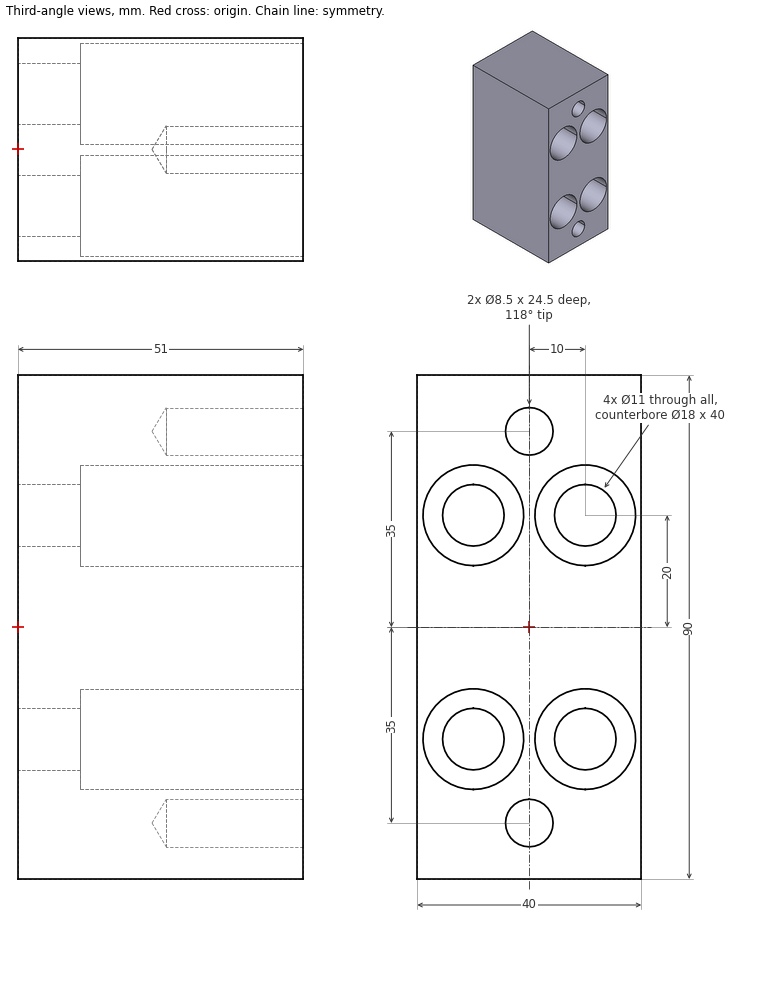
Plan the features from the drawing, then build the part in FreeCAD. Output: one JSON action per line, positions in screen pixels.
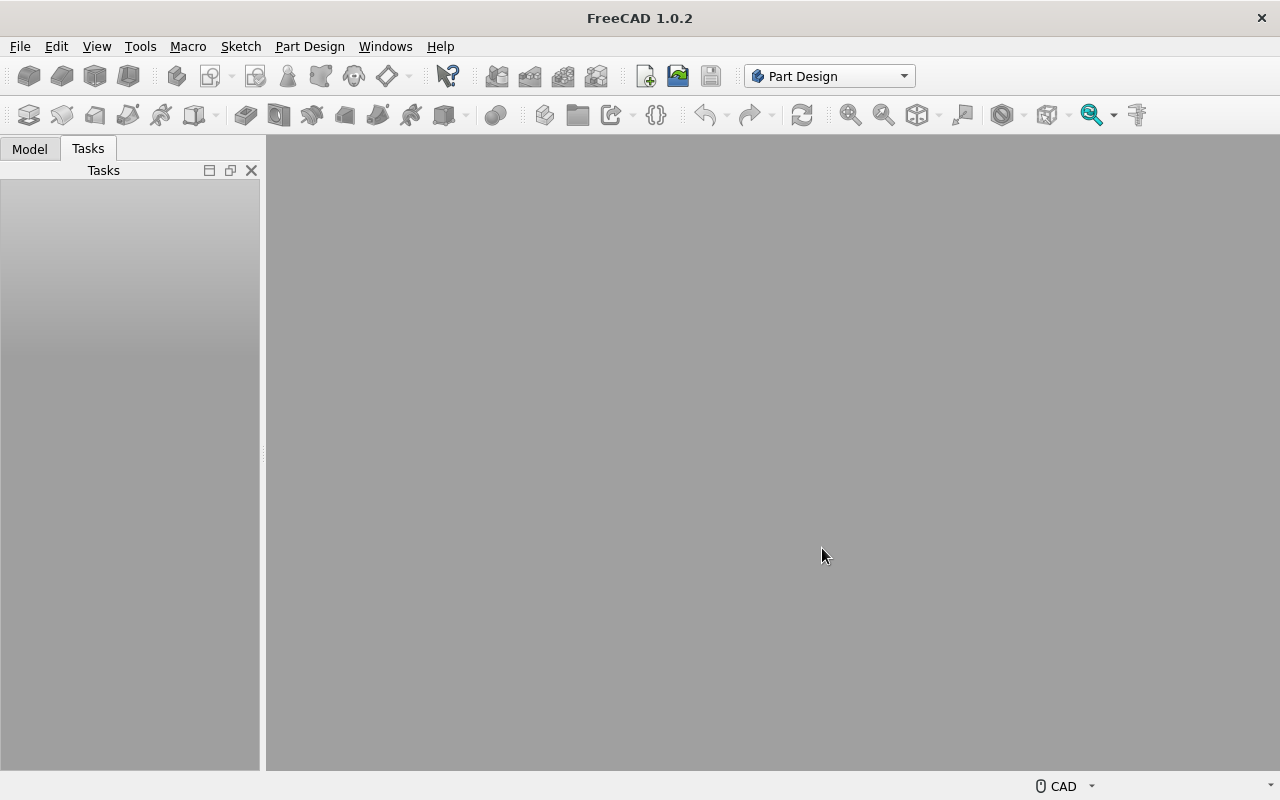
{"action": "left_click", "coordinate": [645, 76]}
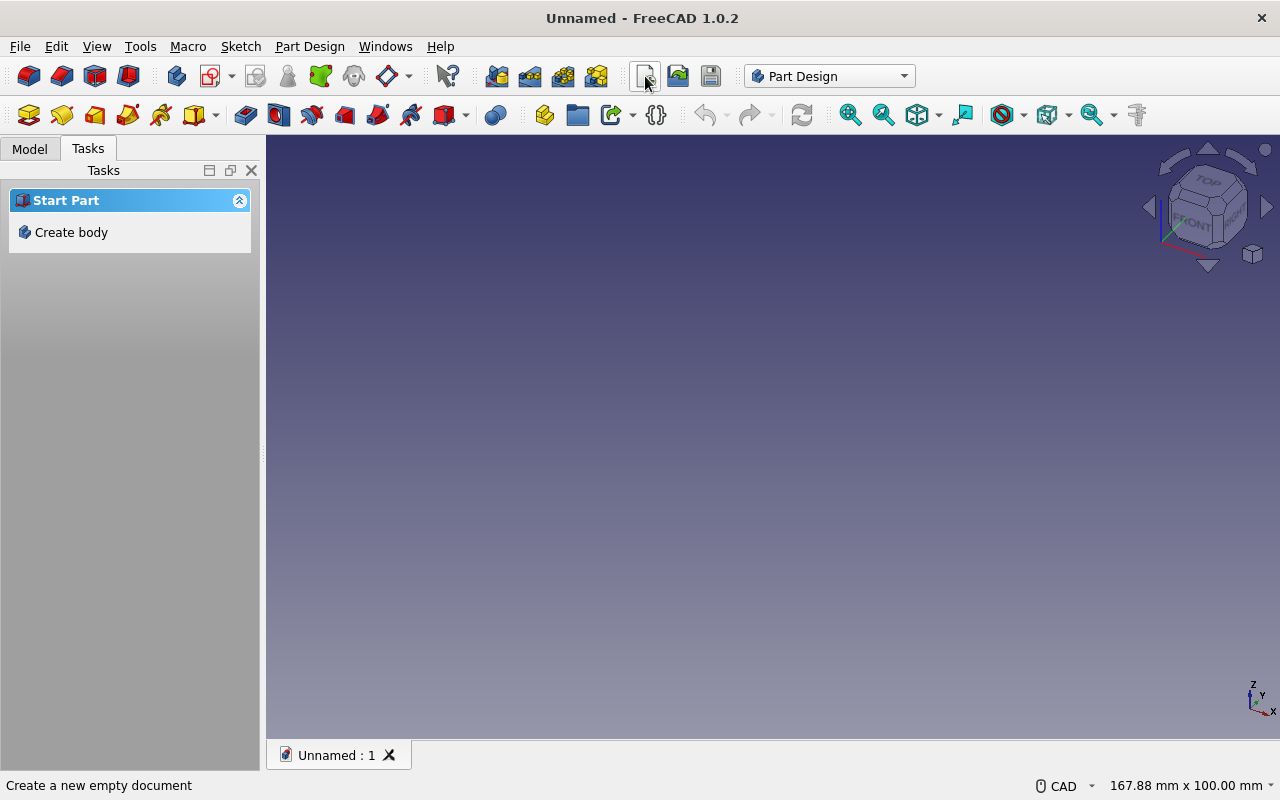
{"action": "left_click", "coordinate": [210, 76]}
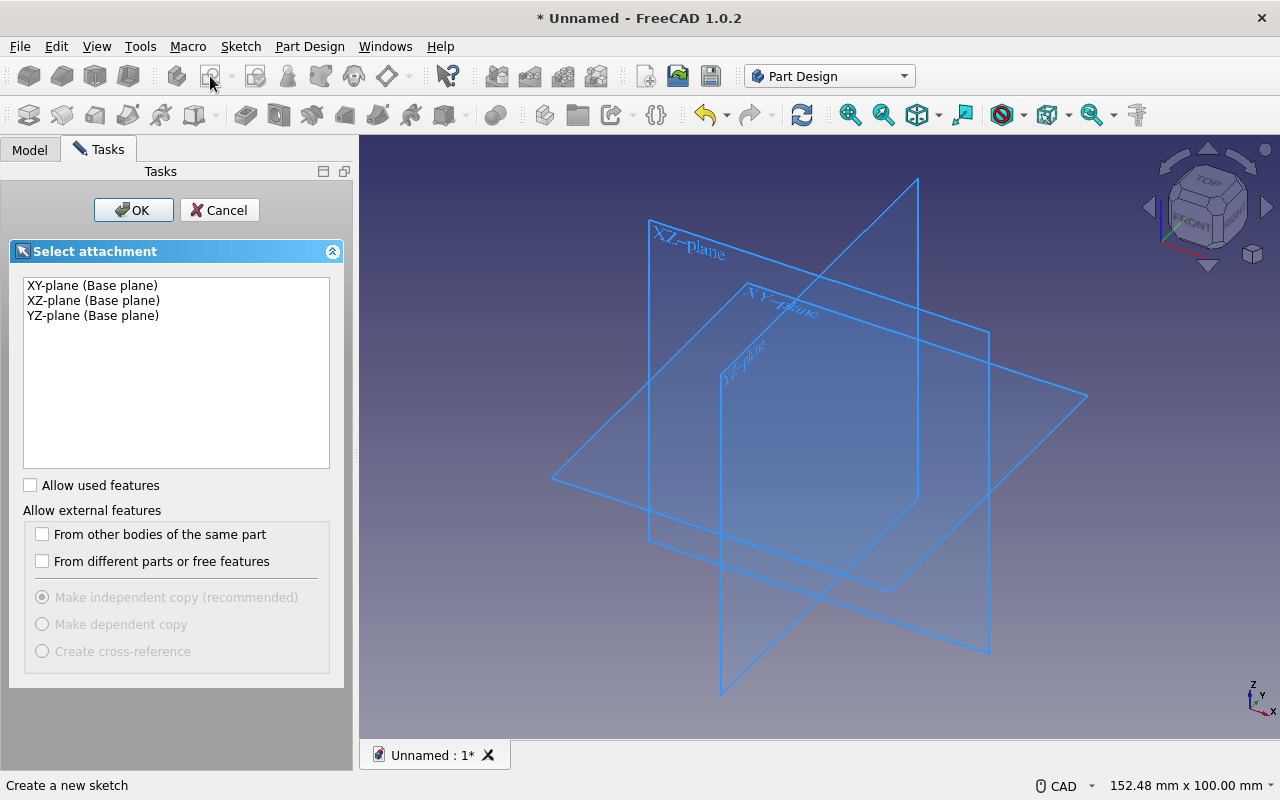
{"action": "left_click", "coordinate": [84, 316]}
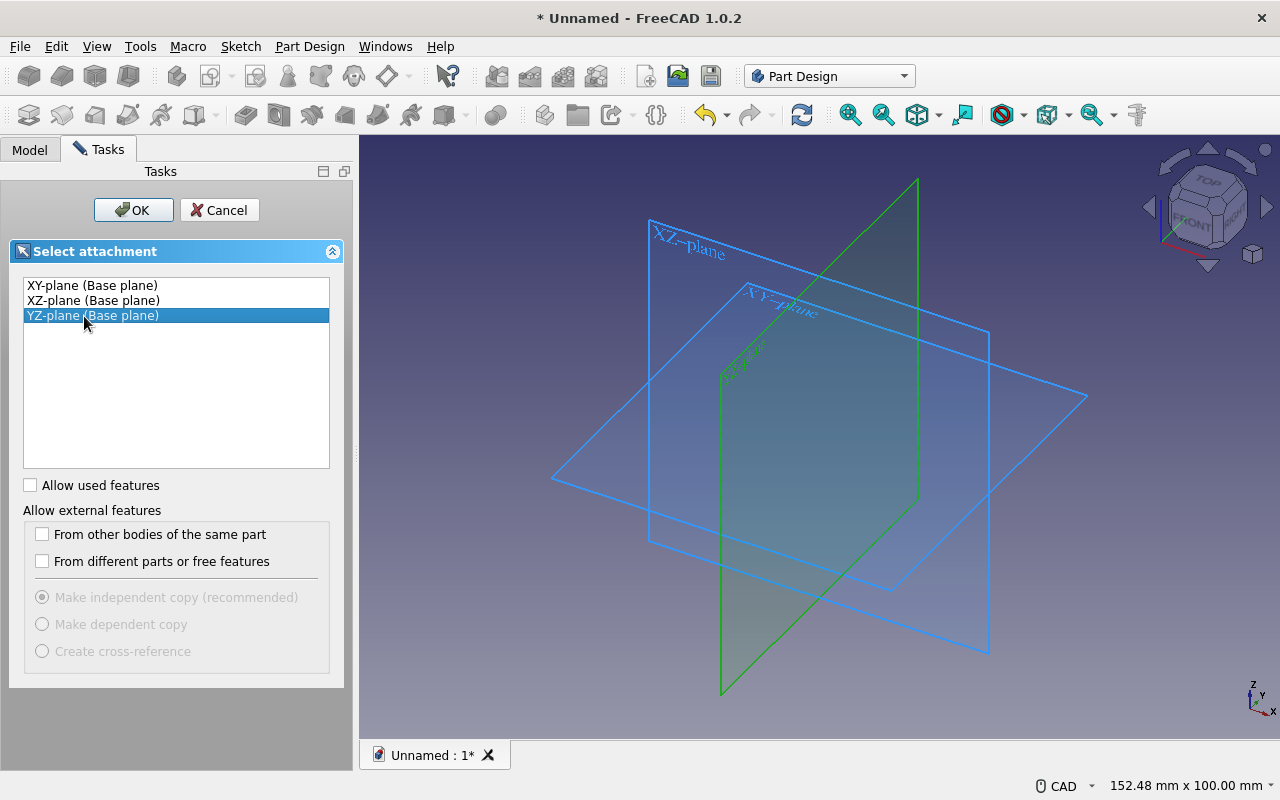
{"action": "left_click", "coordinate": [134, 210]}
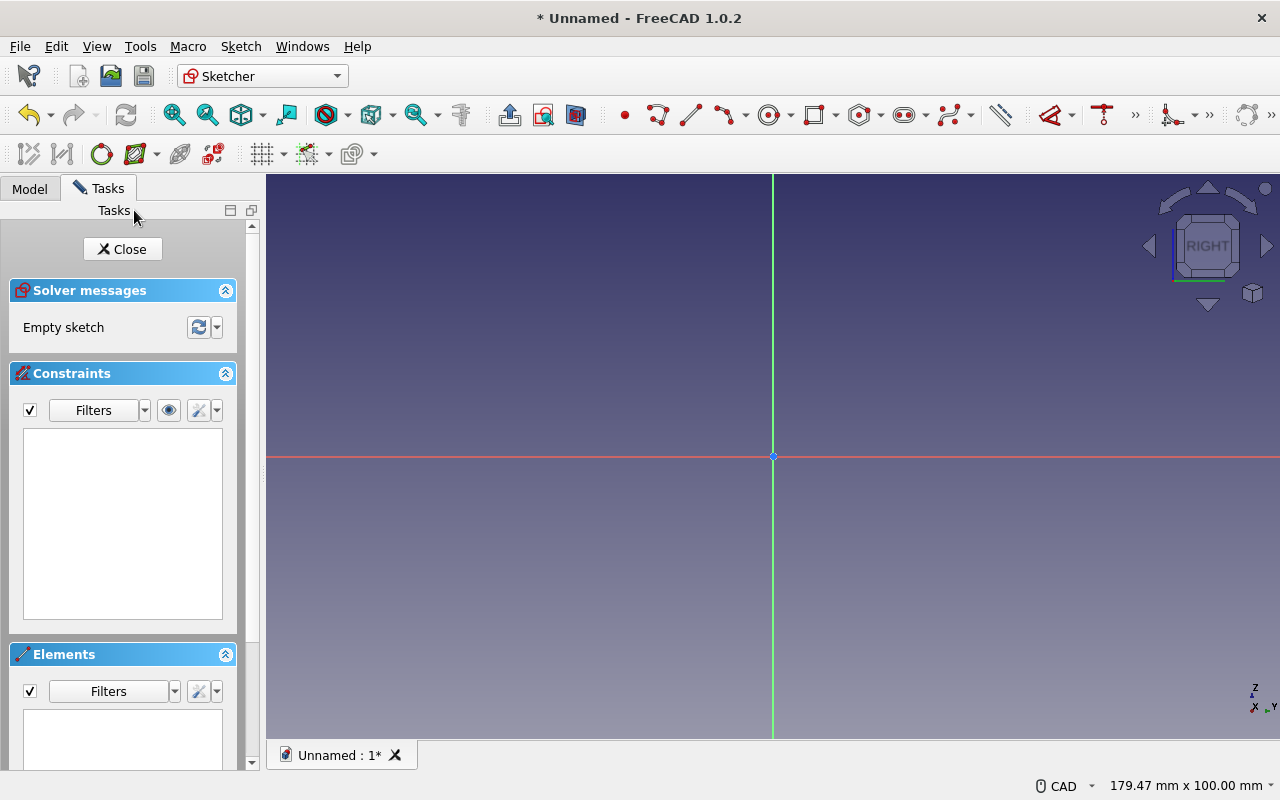
{"action": "scroll", "coordinate": [565, 457], "scroll_direction": "down", "scroll_amount": 2}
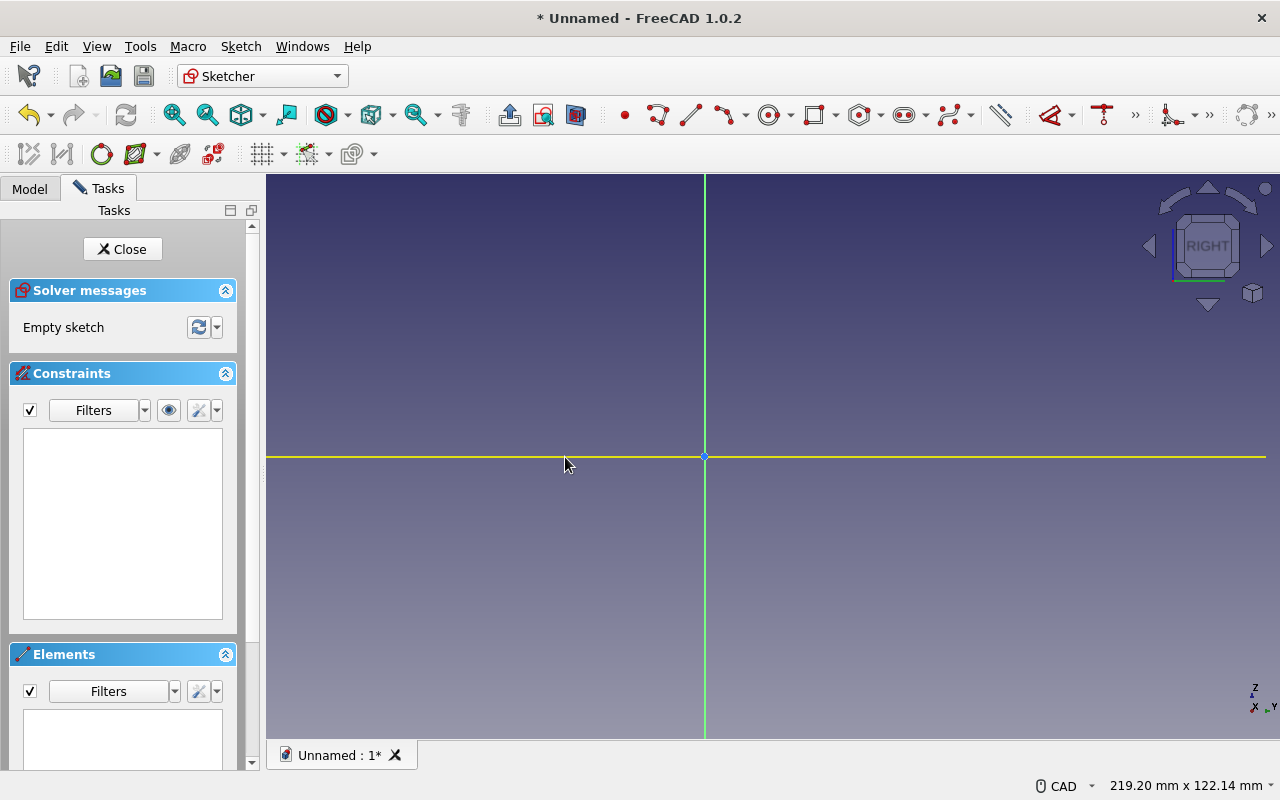
{"action": "key", "text": "g v"}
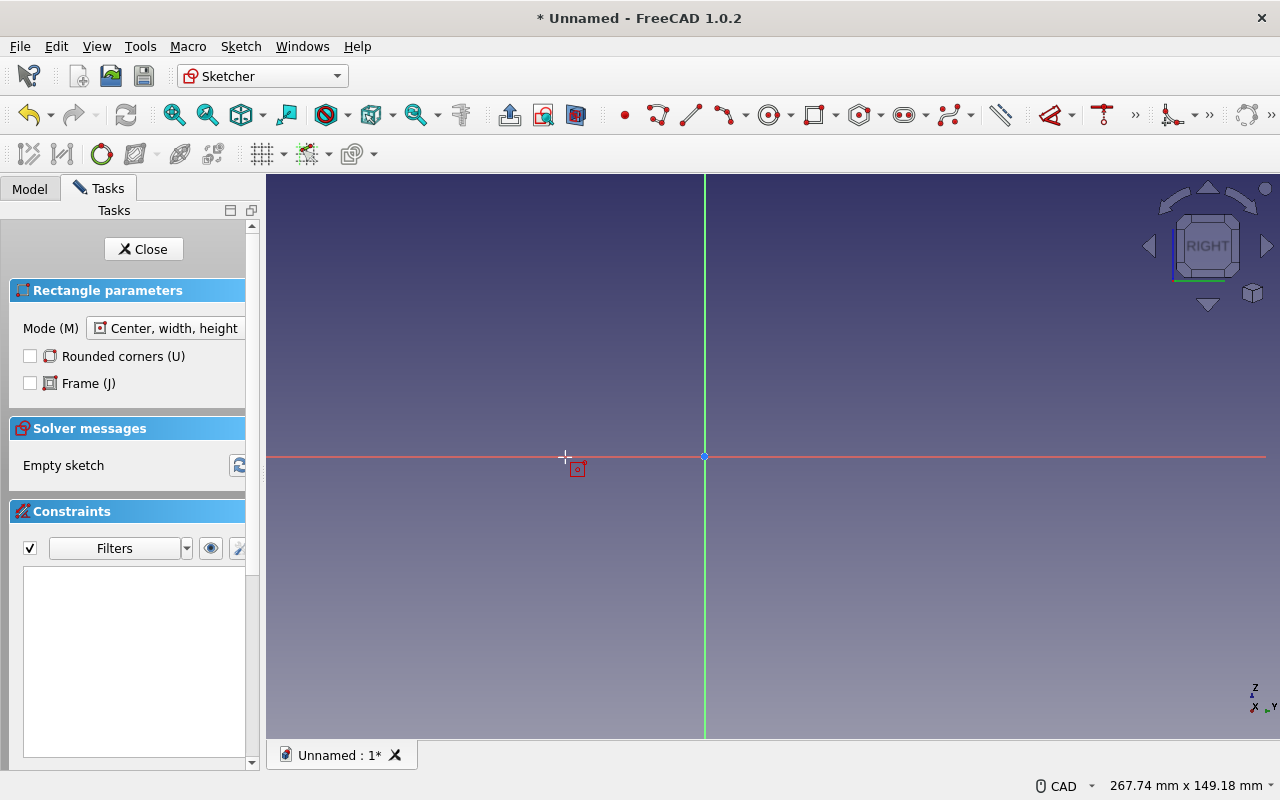
{"action": "left_click", "coordinate": [705, 457]}
{"action": "mouse_move", "coordinate": [780, 286]}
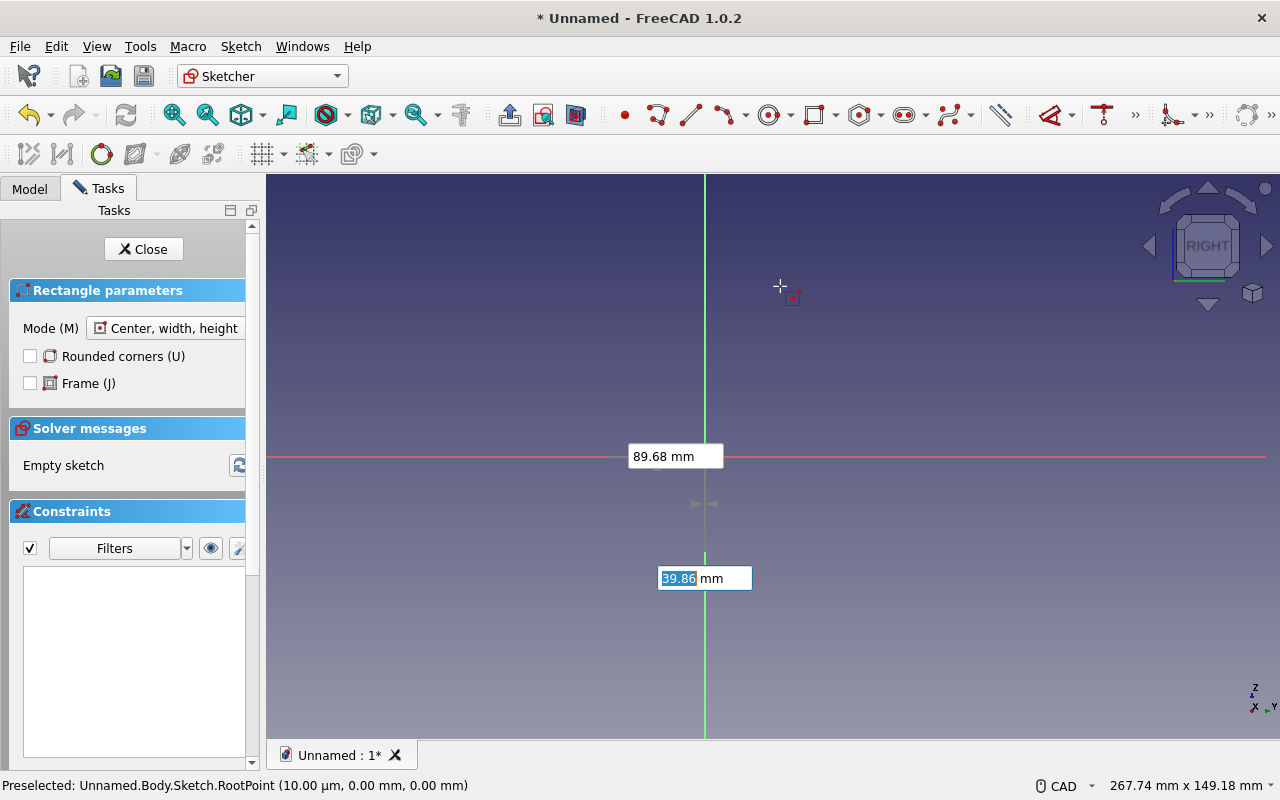
{"action": "type", "text": "40"}
{"action": "key", "text": "Tab"}
{"action": "type", "text": "90"}
{"action": "key", "text": "Return"}
{"action": "key", "text": "Escape"}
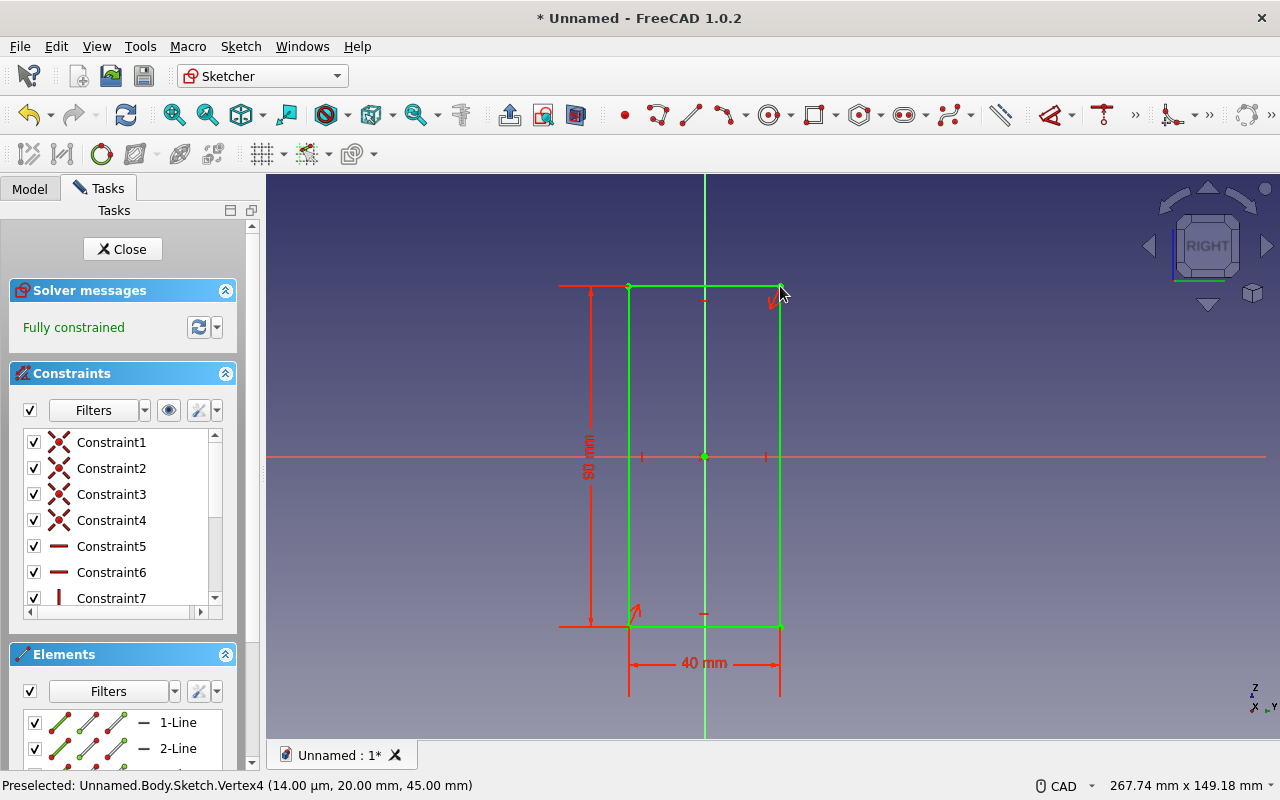
{"action": "left_click", "coordinate": [123, 249]}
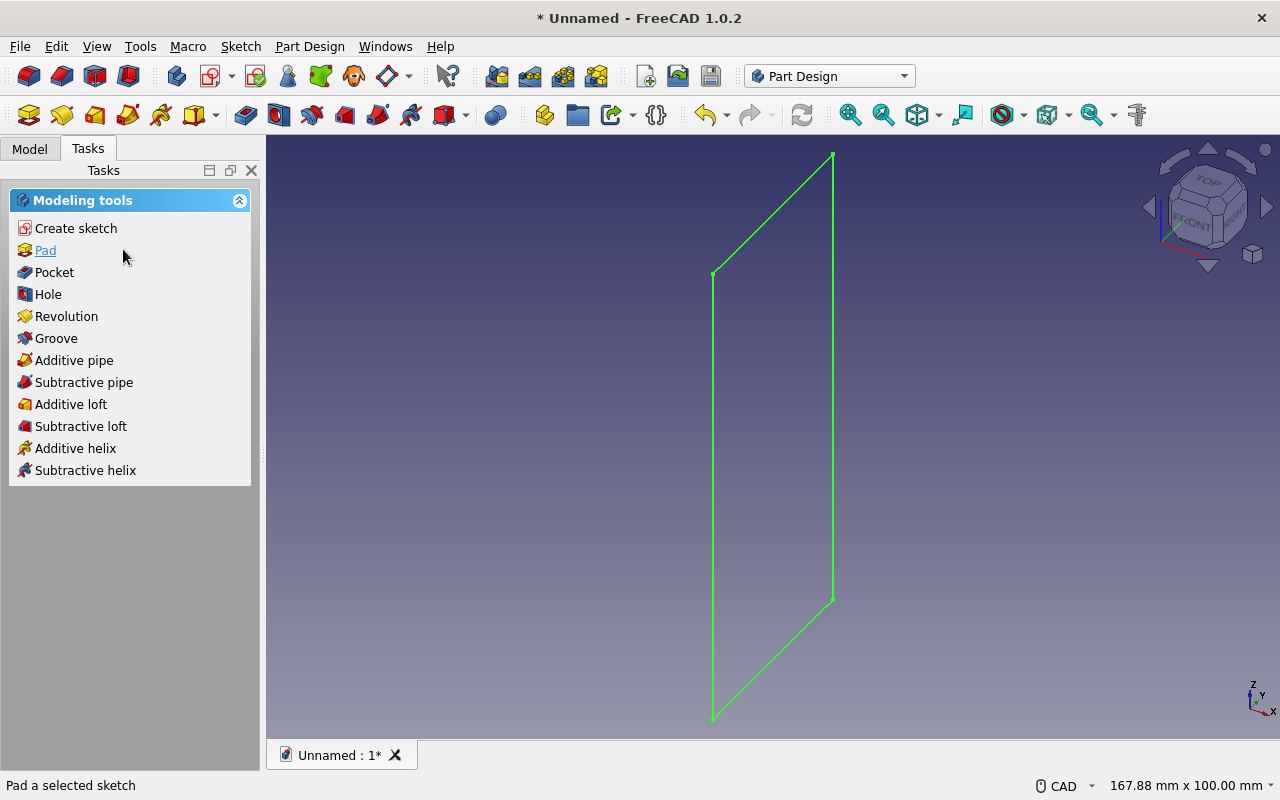
{"action": "left_click", "coordinate": [29, 116]}